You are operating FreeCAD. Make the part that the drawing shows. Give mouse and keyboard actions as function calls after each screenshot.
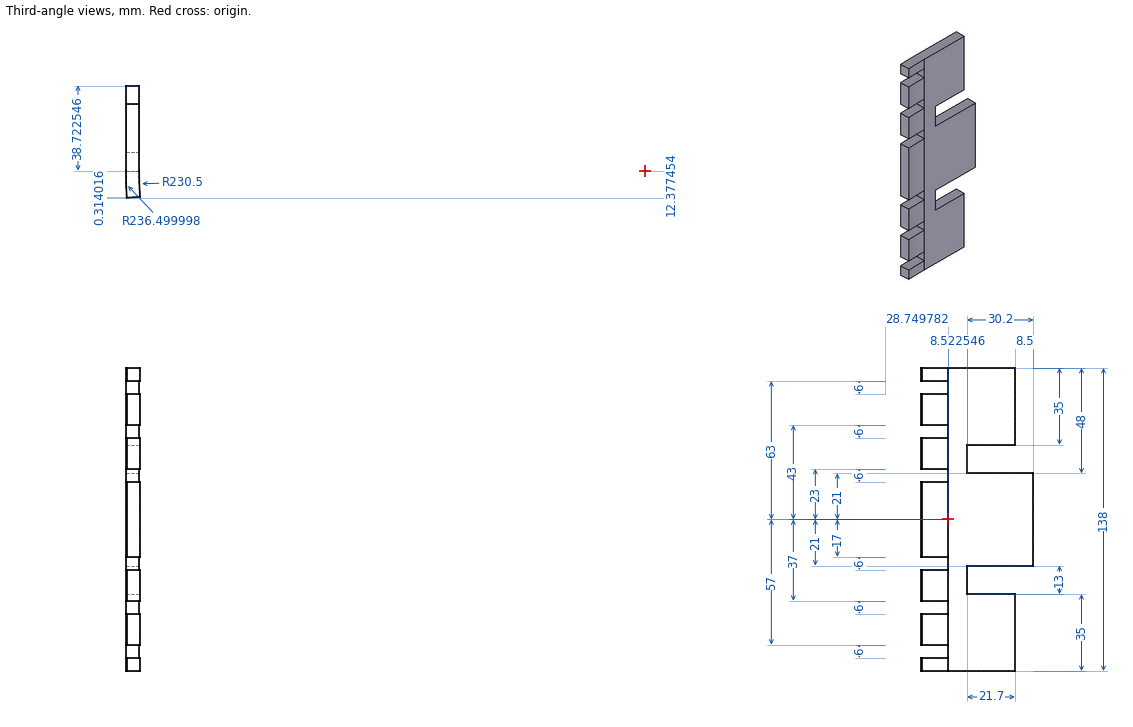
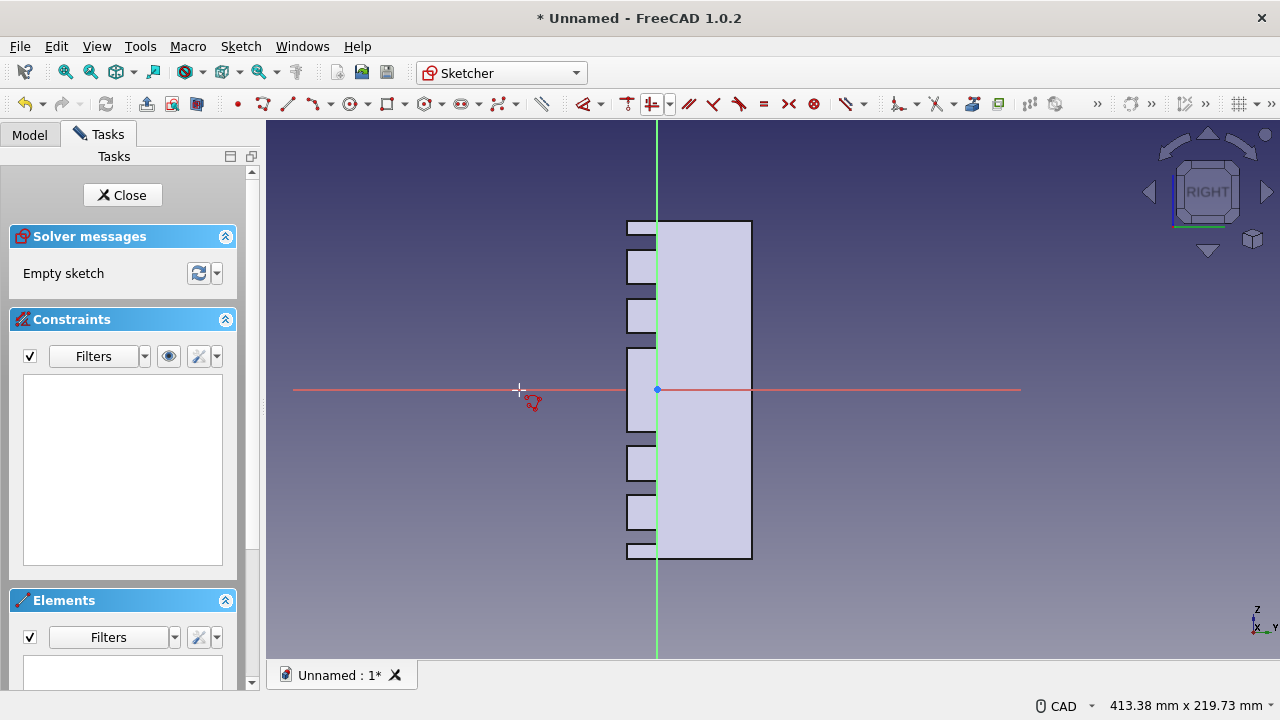
click(678, 338)
click(752, 338)
click(752, 221)
click(731, 221)
click(731, 306)
click(678, 306)
click(678, 339)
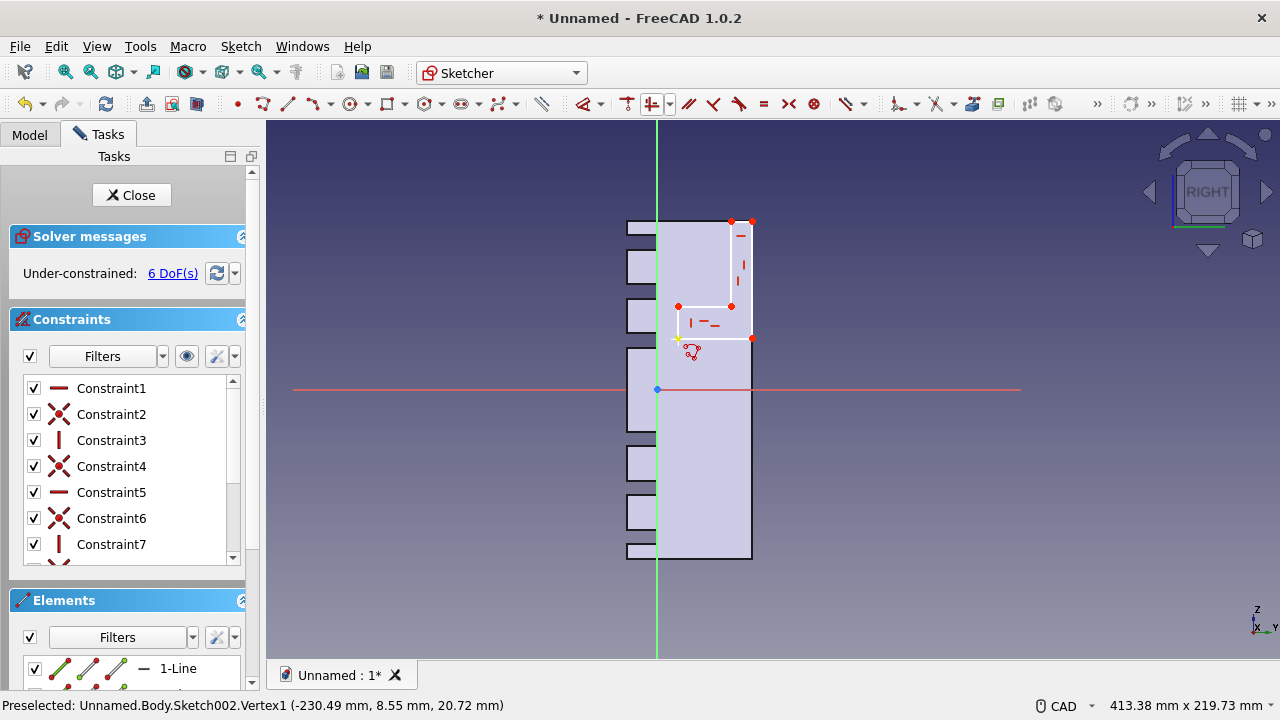
click(678, 441)
click(678, 473)
click(731, 473)
click(731, 559)
click(752, 559)
click(752, 441)
click(678, 442)
key(Escape)
key(Escape)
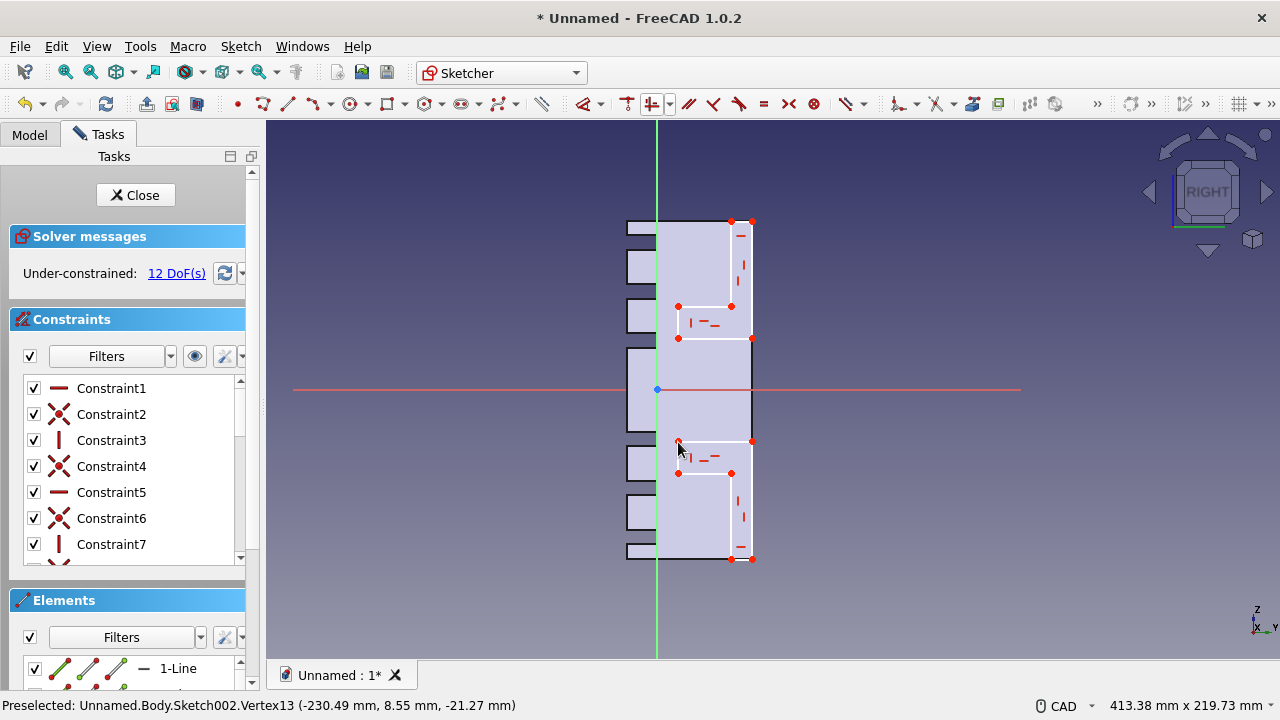
click(582, 104)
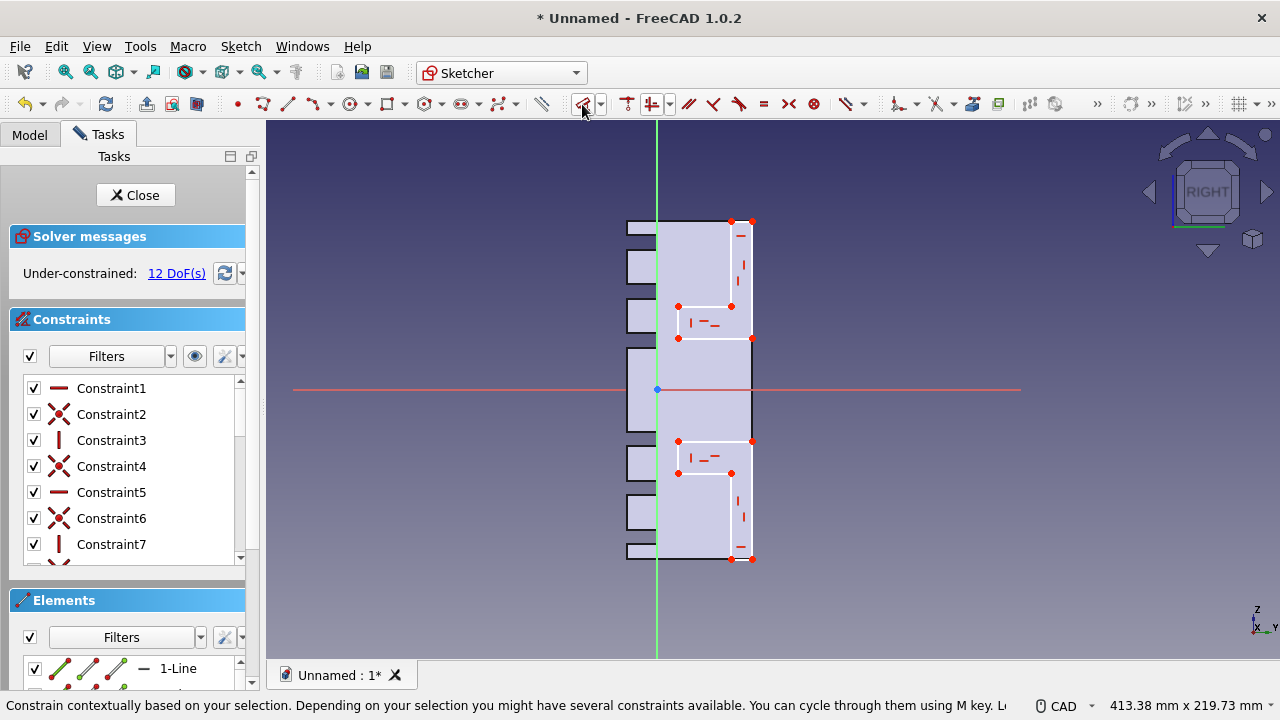
click(752, 304)
click(786, 281)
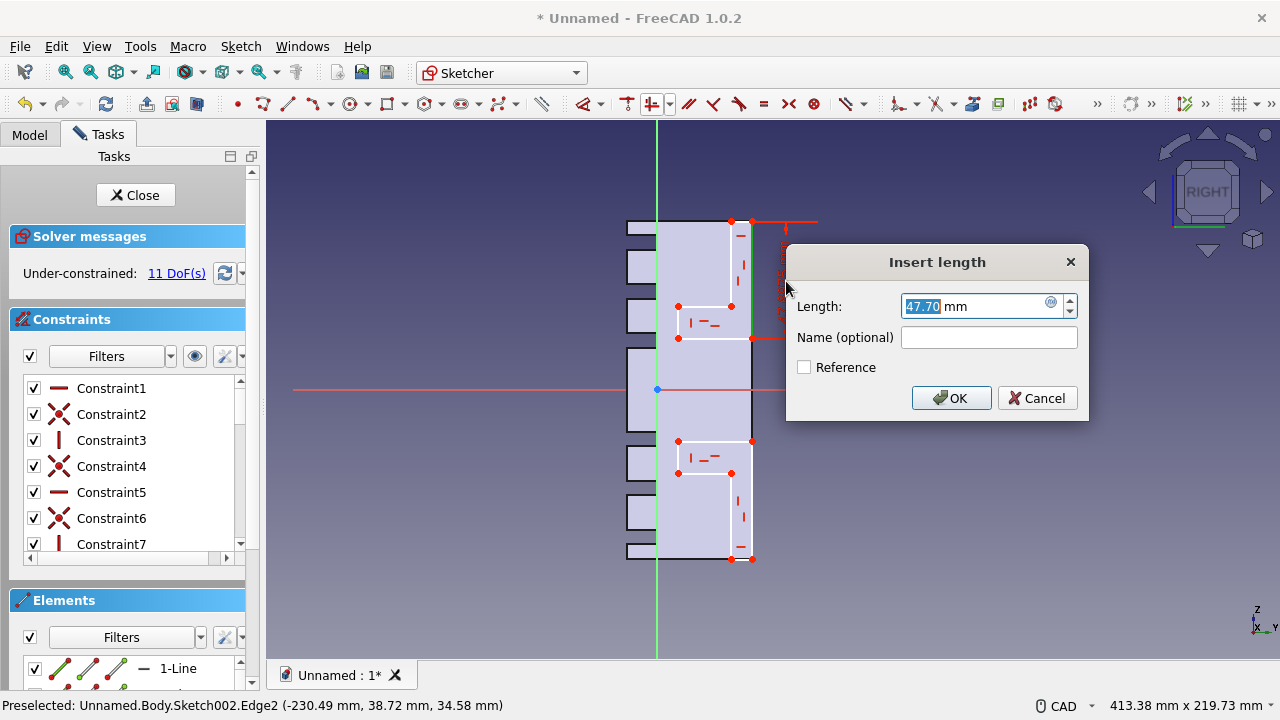
text(48)
key(Return)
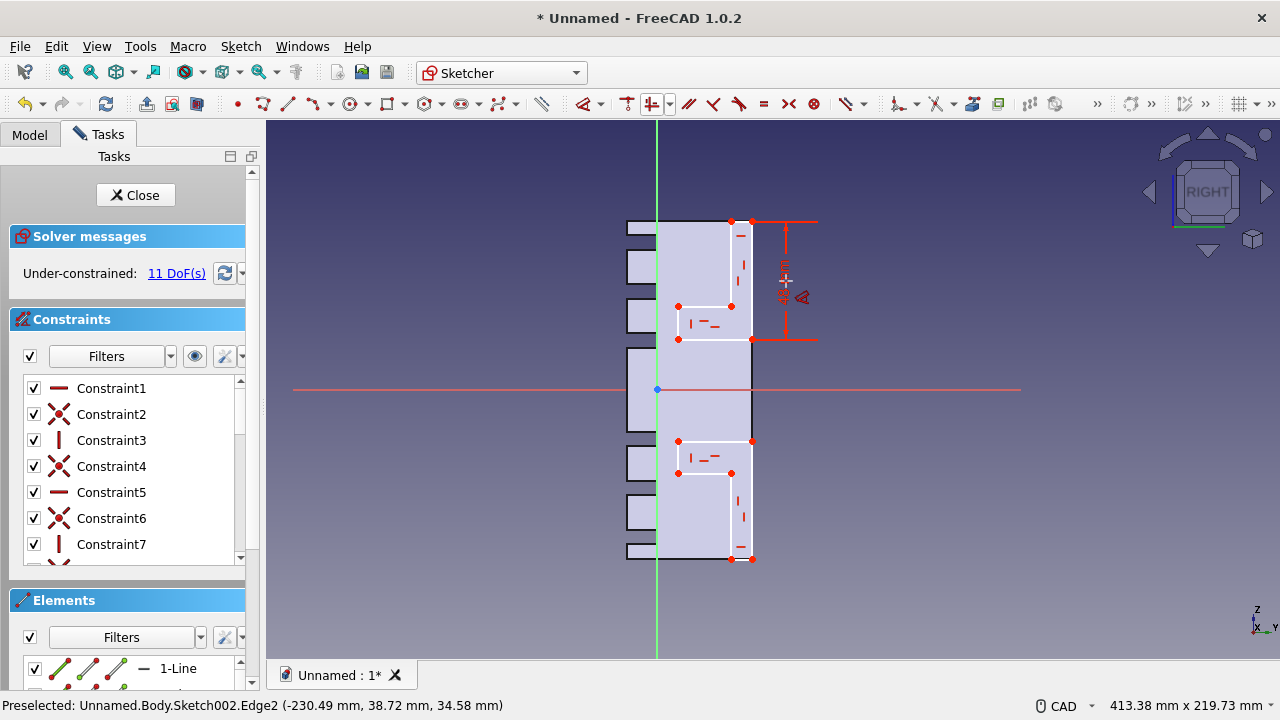
click(731, 247)
click(697, 264)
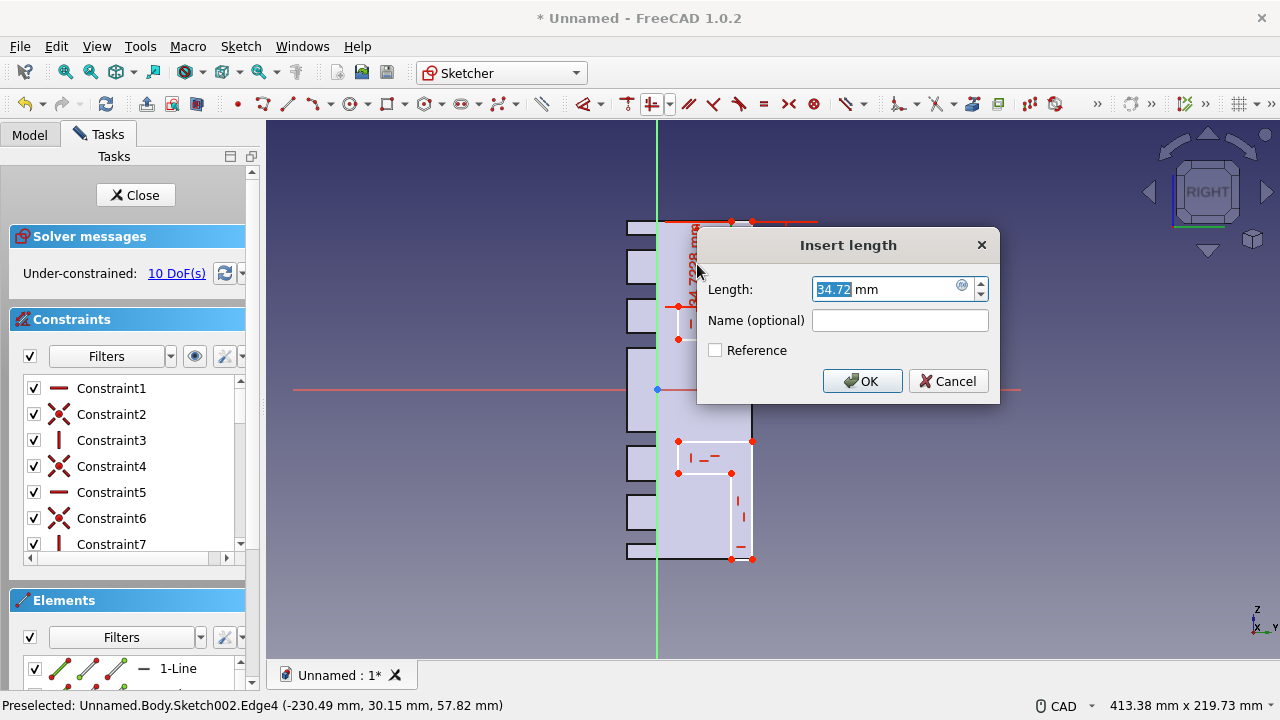
text(35)
key(Return)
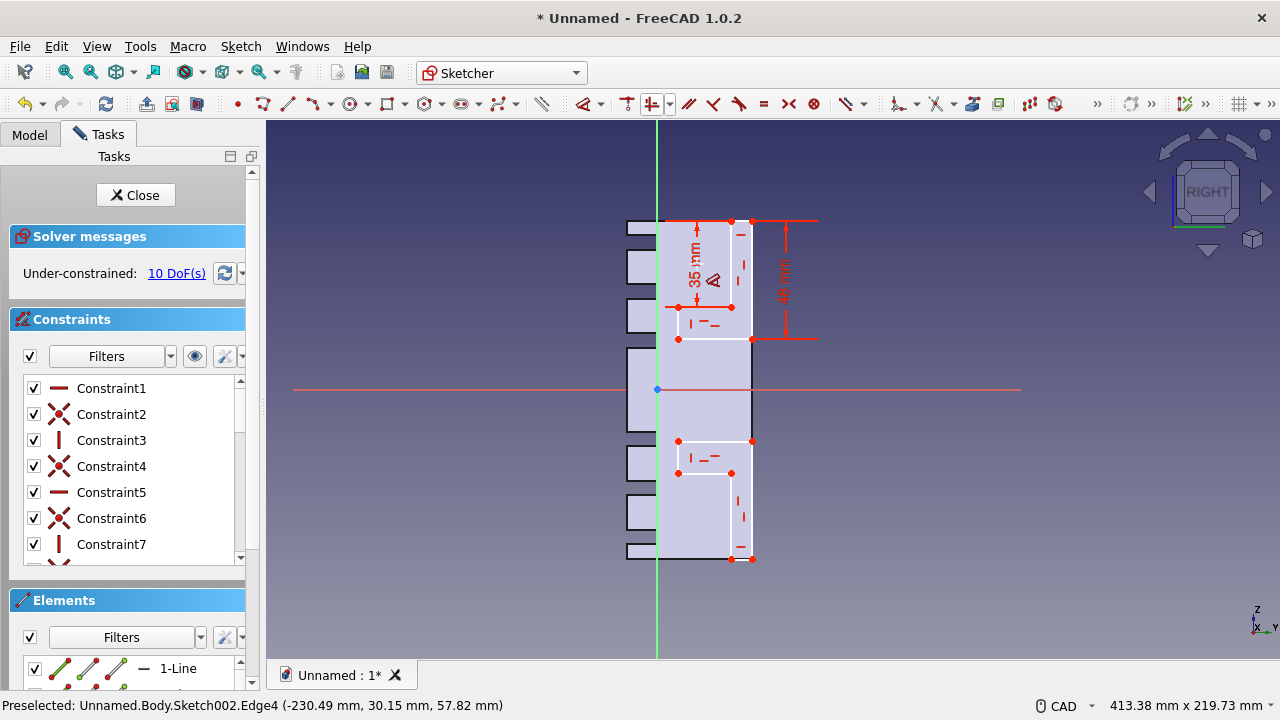
scroll(678, 452, up, 2)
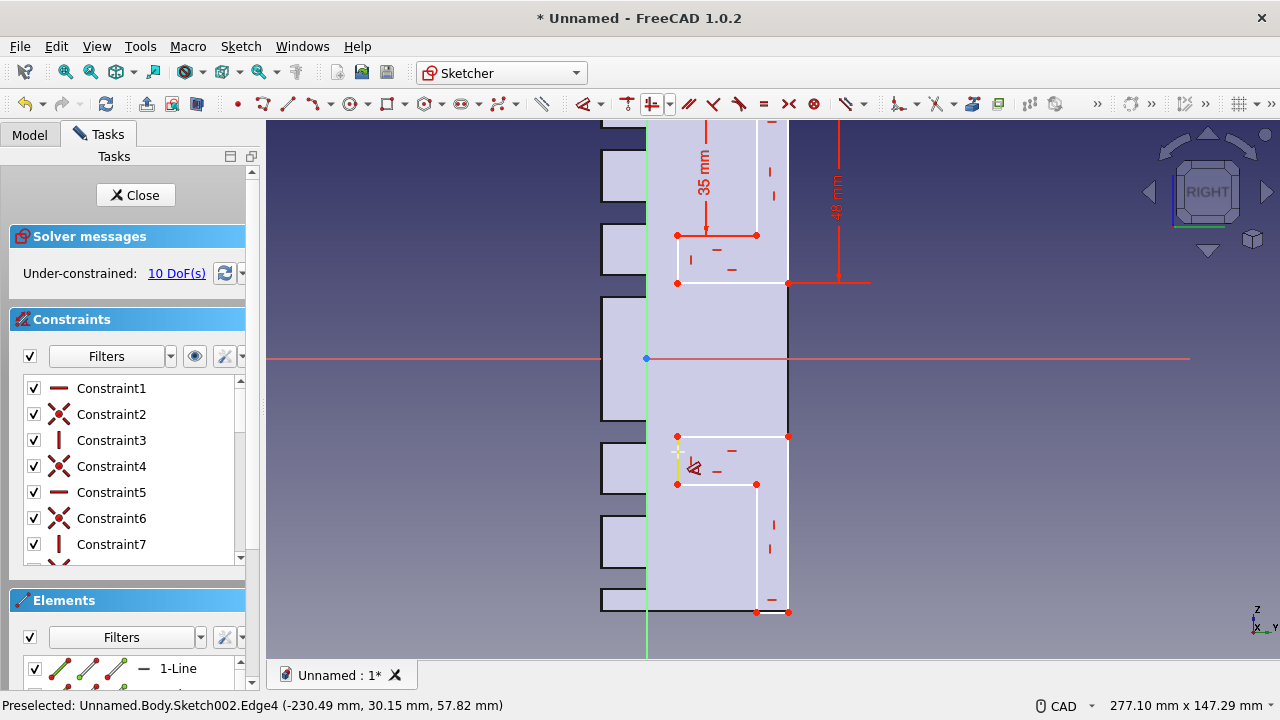
click(678, 451)
click(712, 461)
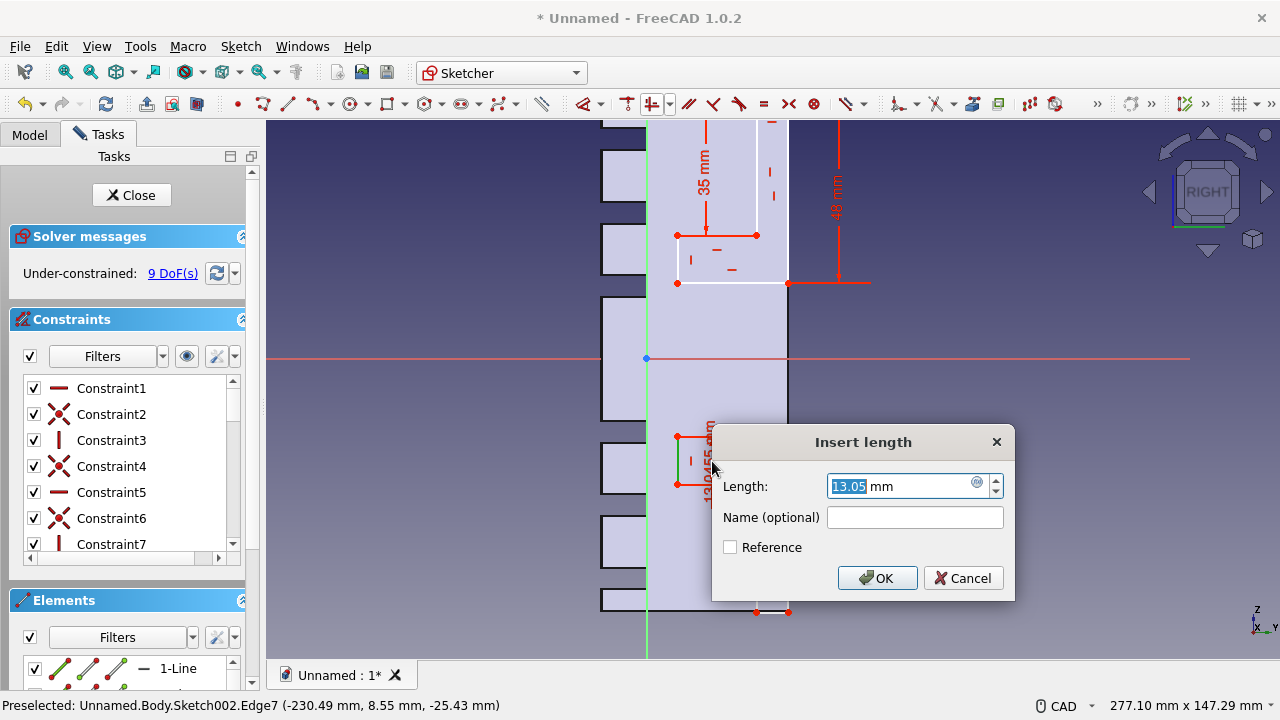
text(13)
key(Return)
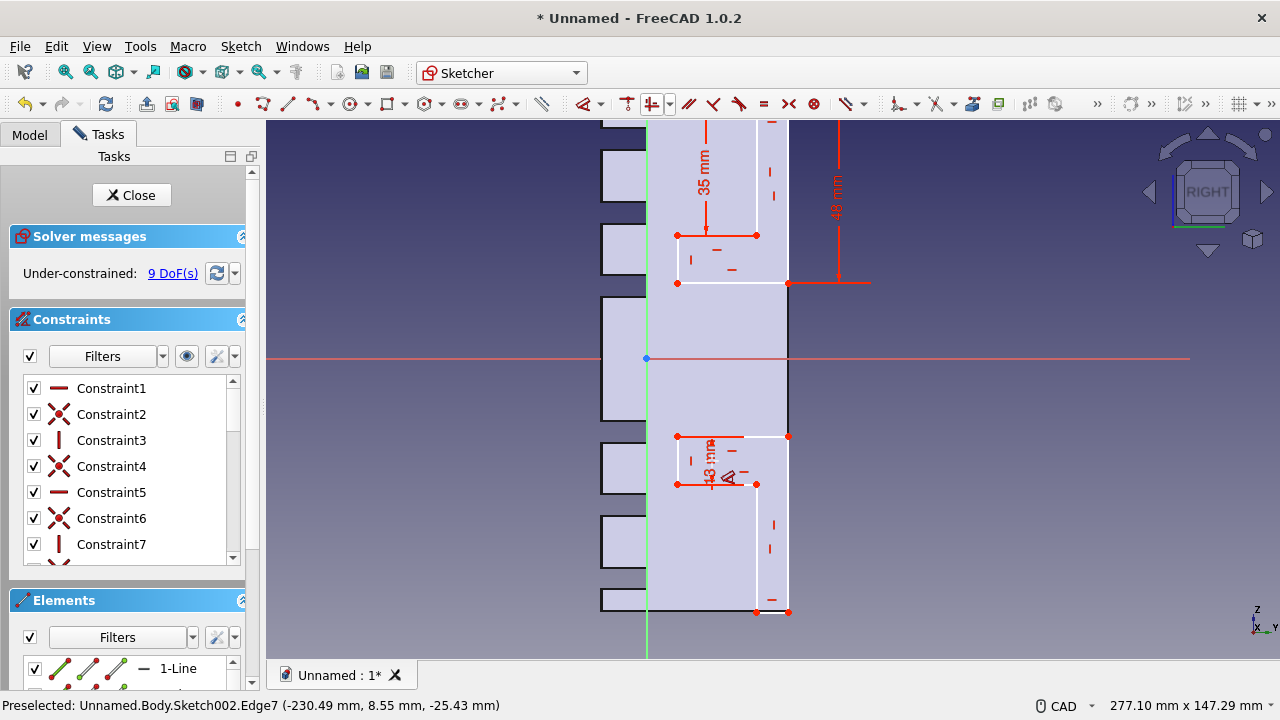
click(757, 523)
click(723, 549)